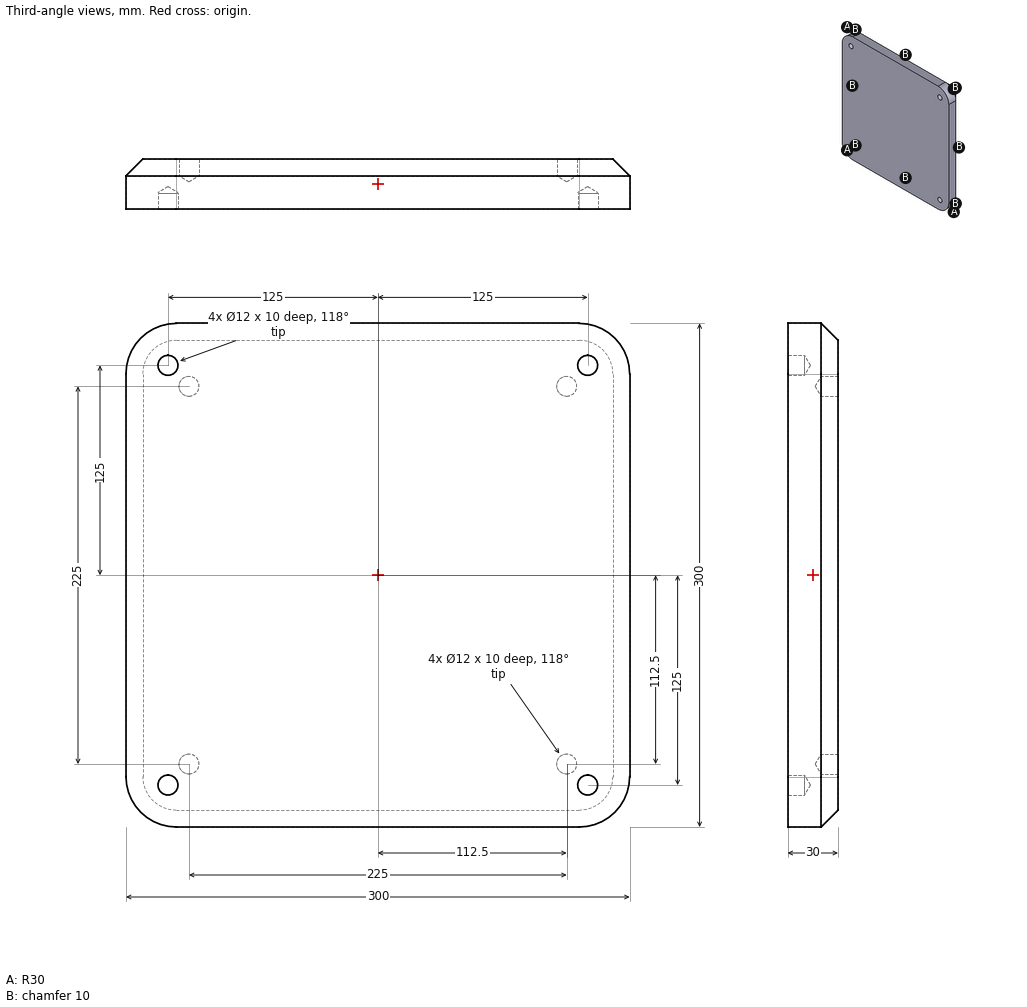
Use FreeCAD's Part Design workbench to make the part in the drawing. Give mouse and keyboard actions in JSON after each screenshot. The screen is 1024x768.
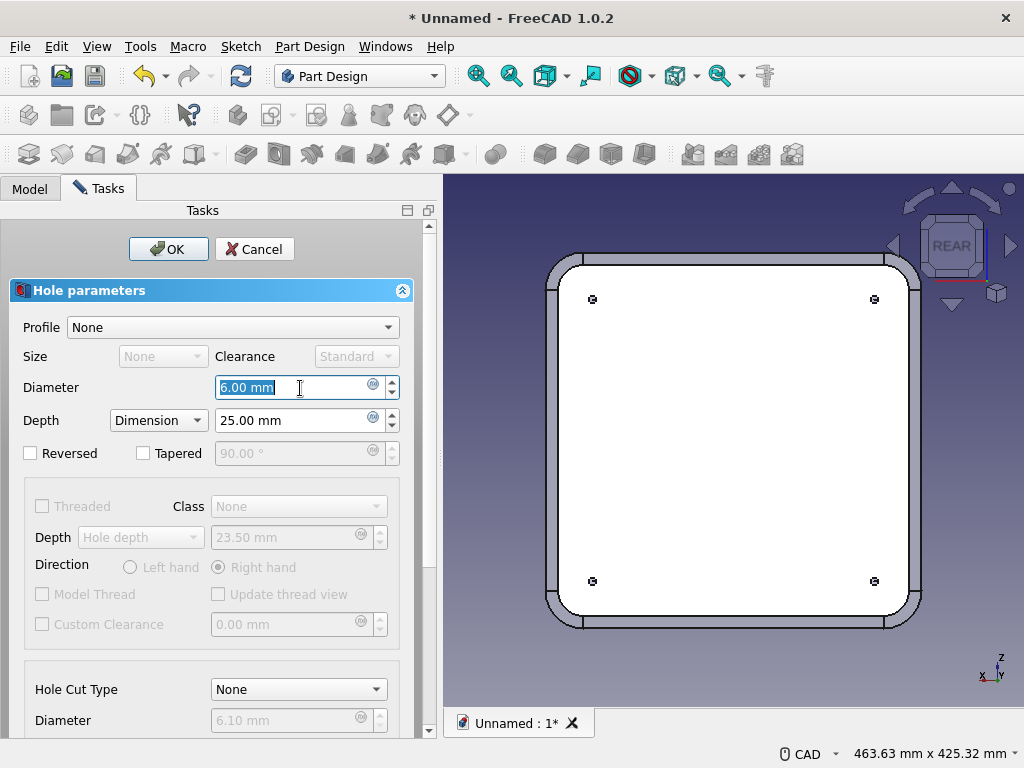
{"action": "type", "text": "12"}
{"action": "key", "text": "Tab"}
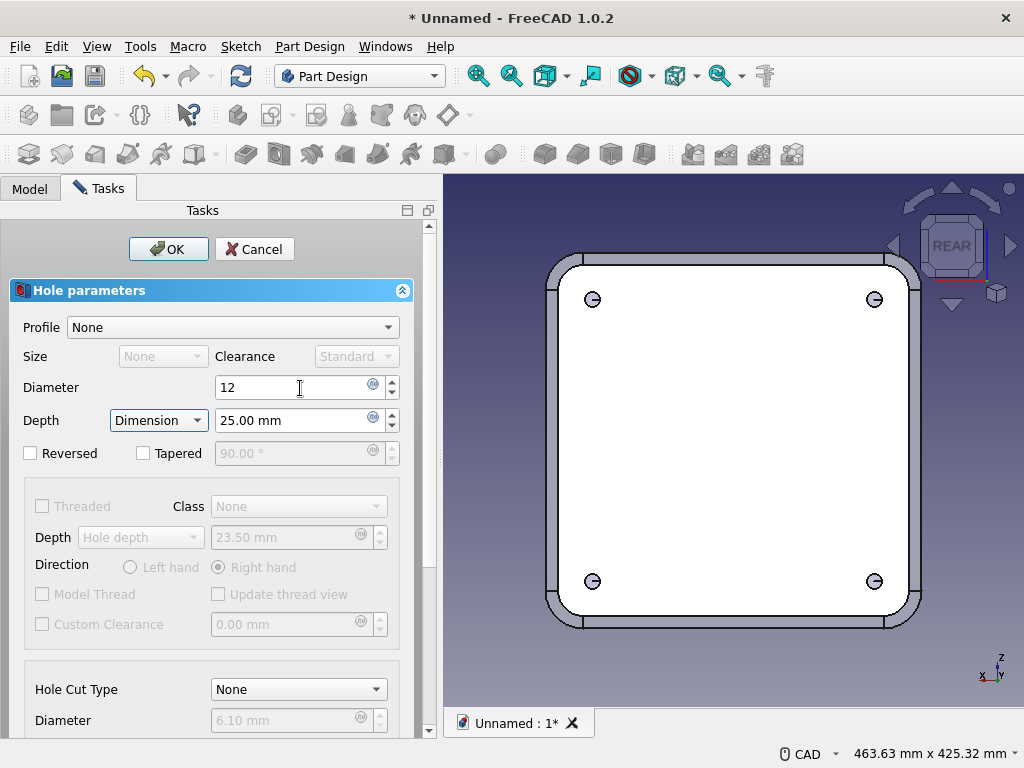
{"action": "triple_click", "coordinate": [300, 420]}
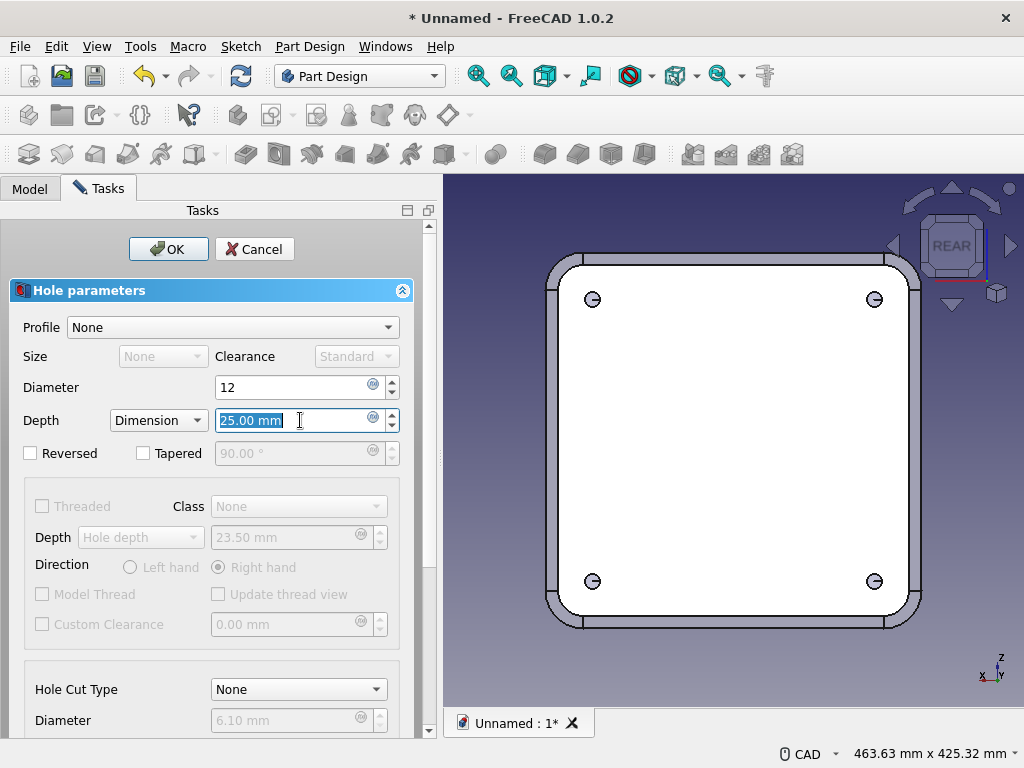
{"action": "type", "text": "10"}
{"action": "key", "text": "Tab"}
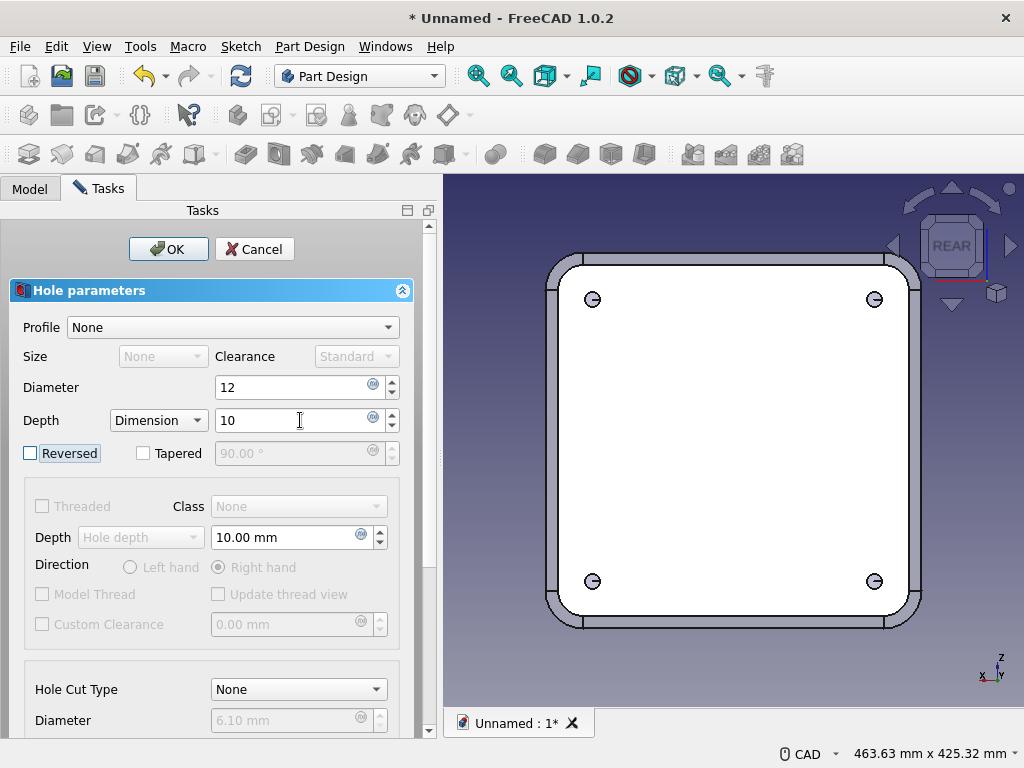
{"action": "left_click", "coordinate": [169, 249]}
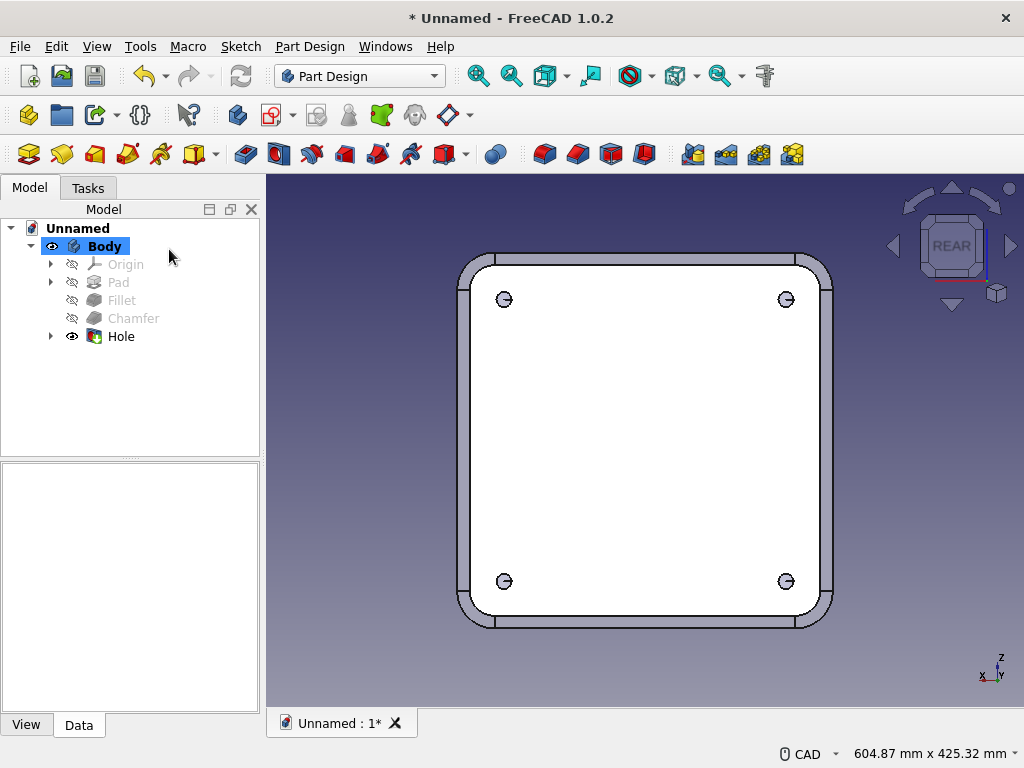
{"action": "key", "text": "0"}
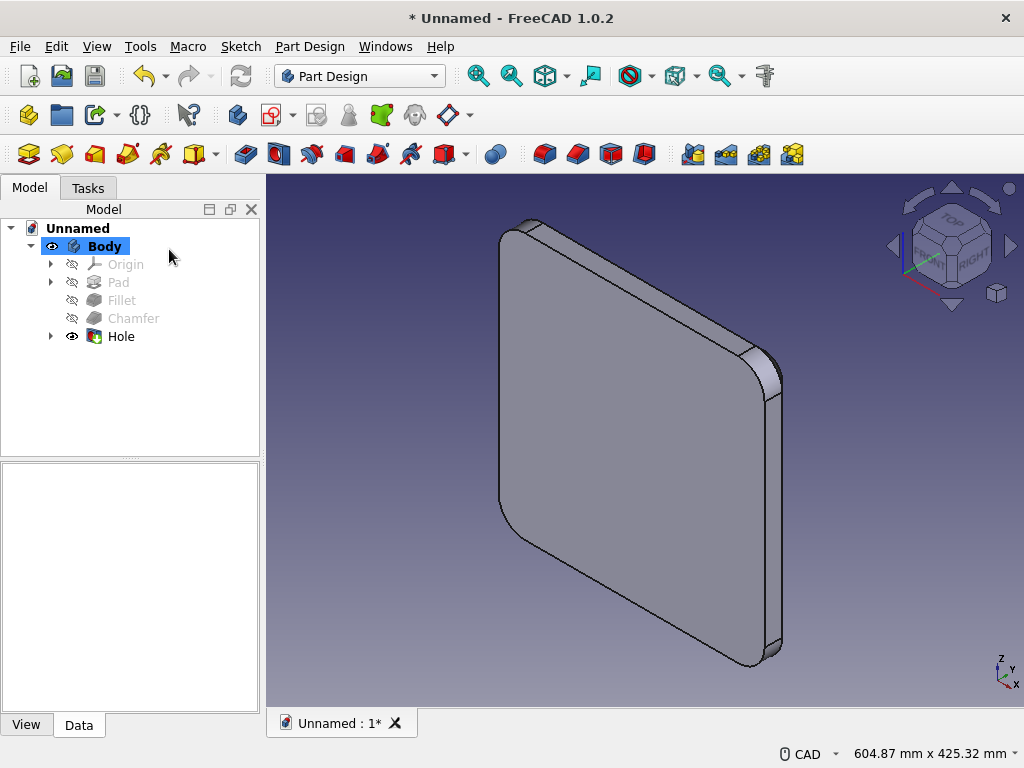
{"action": "left_click", "coordinate": [632, 447]}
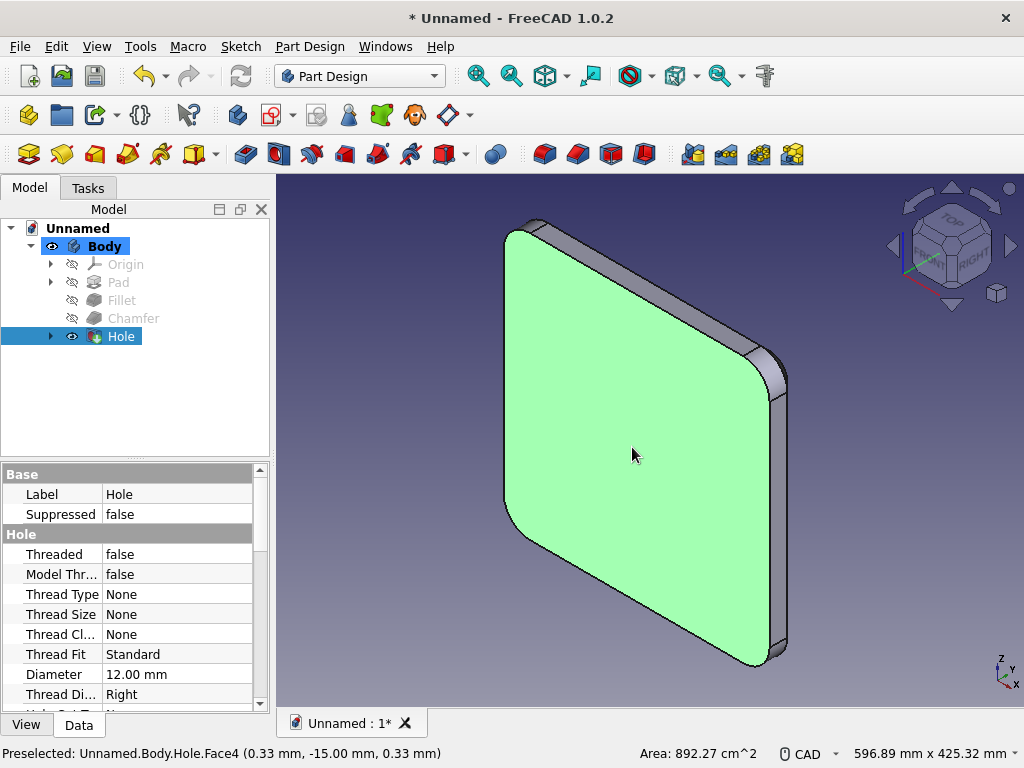
{"action": "left_click", "coordinate": [270, 116]}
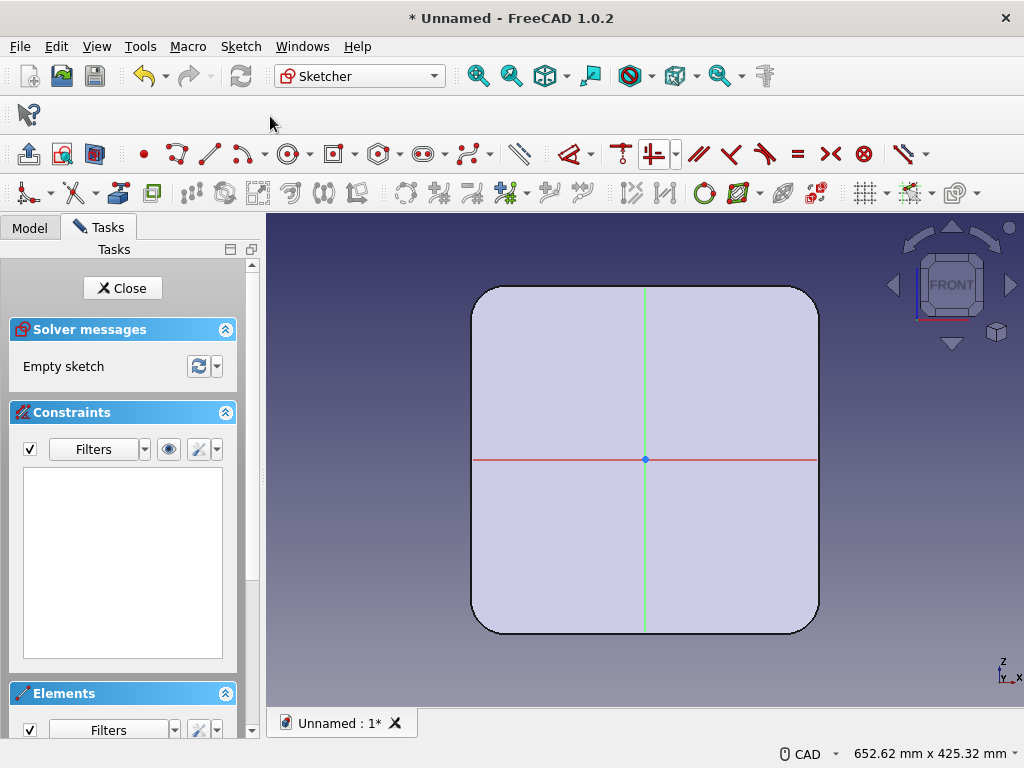
{"action": "left_click", "coordinate": [288, 154]}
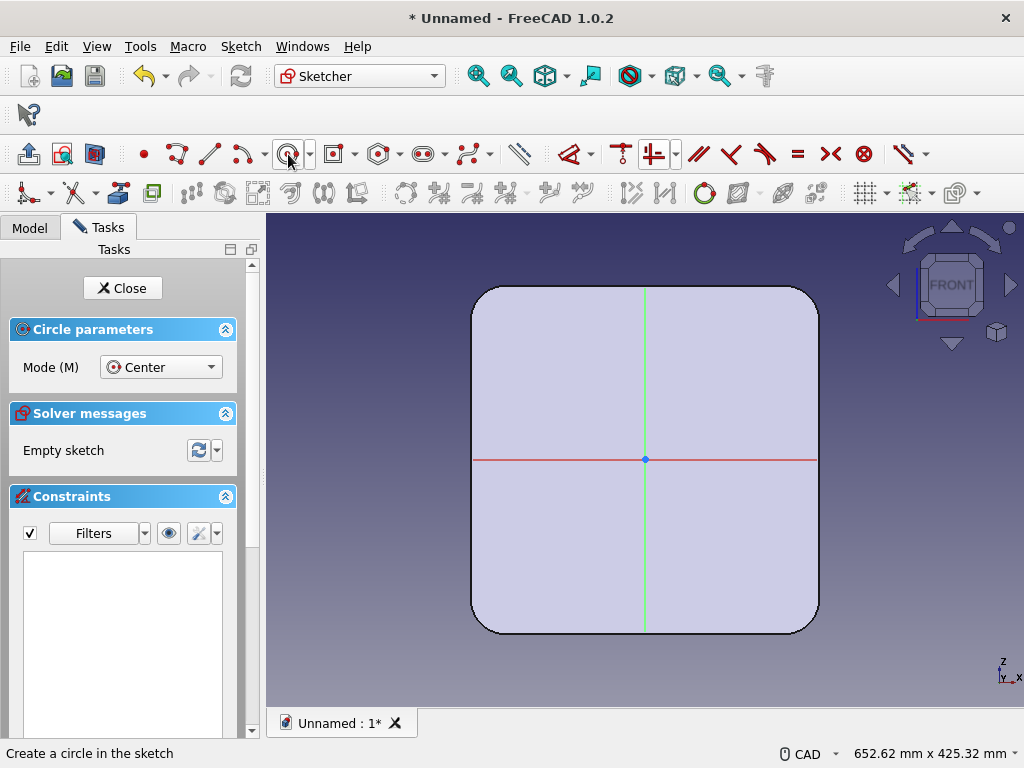
{"action": "scroll", "coordinate": [500, 315], "scroll_direction": "up", "scroll_amount": 6}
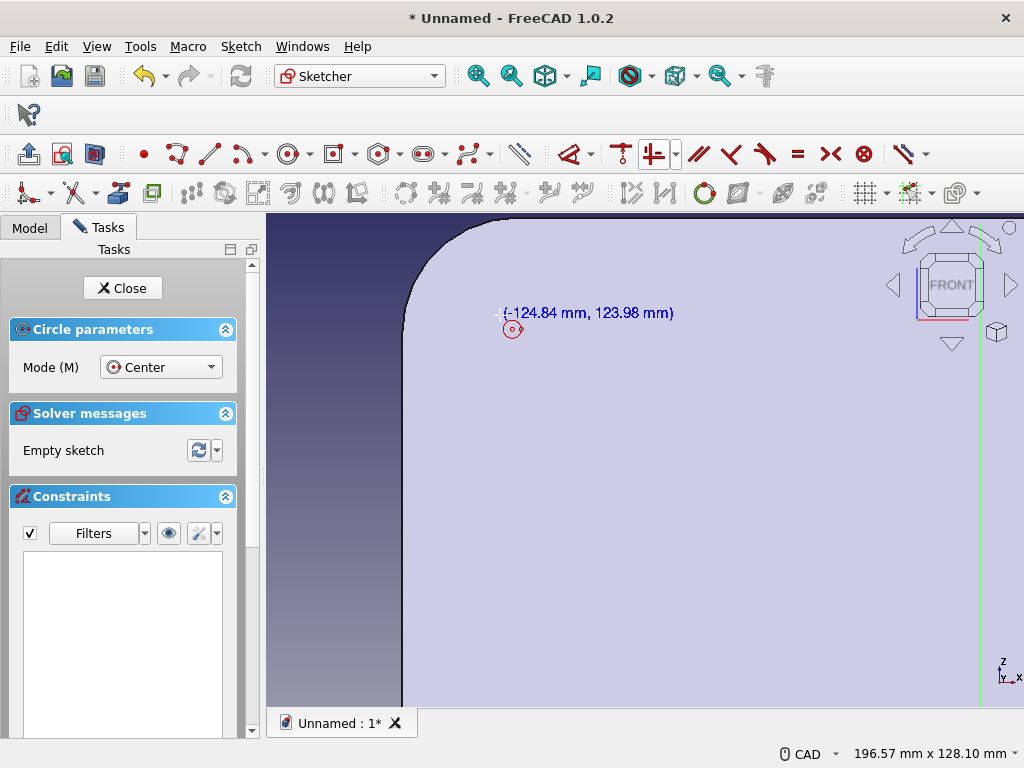
{"action": "left_click", "coordinate": [499, 314]}
{"action": "left_click", "coordinate": [515, 298]}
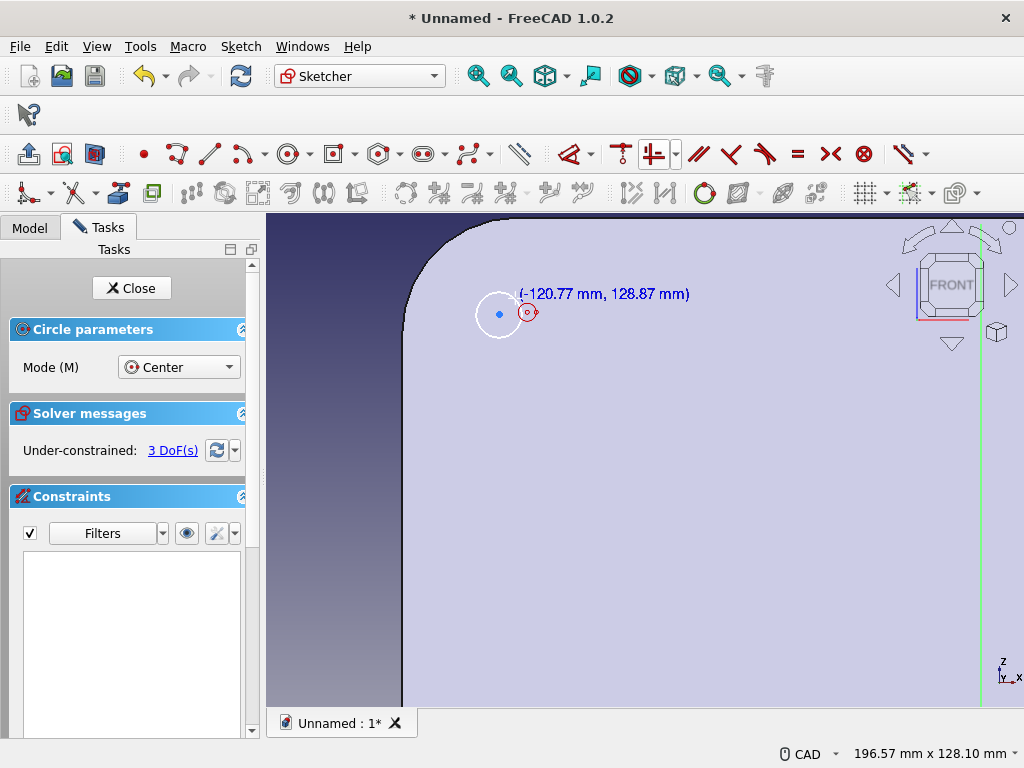
{"action": "scroll", "coordinate": [402, 315], "scroll_direction": "down", "scroll_amount": 6}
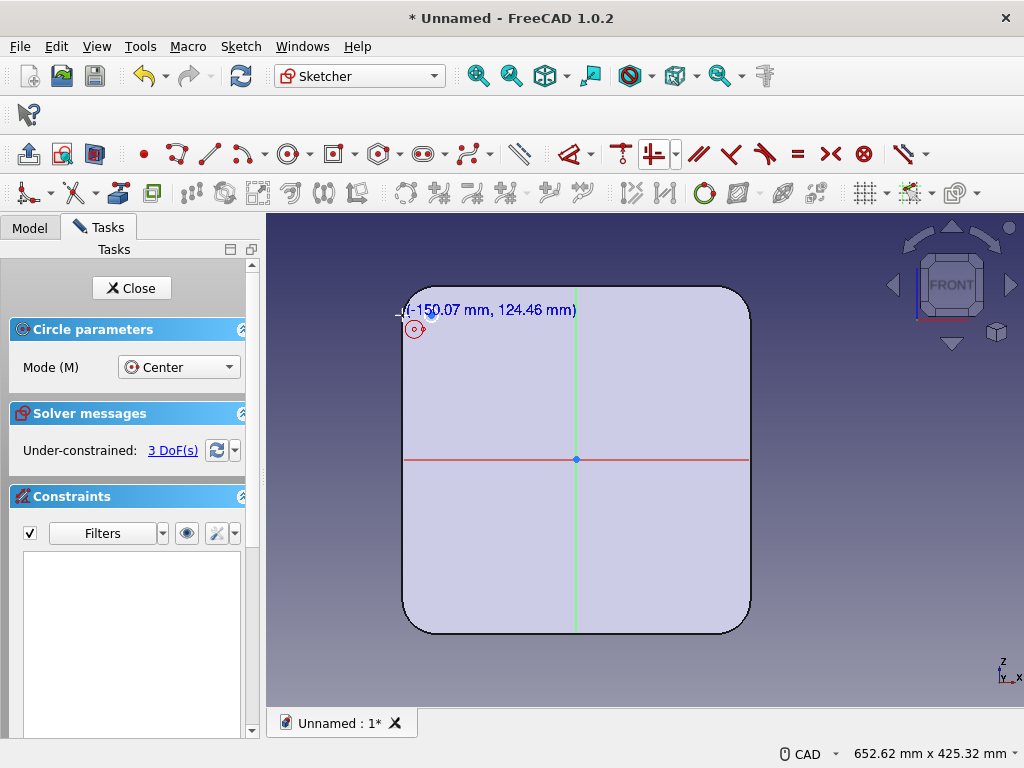
{"action": "scroll", "coordinate": [722, 315], "scroll_direction": "up", "scroll_amount": 6}